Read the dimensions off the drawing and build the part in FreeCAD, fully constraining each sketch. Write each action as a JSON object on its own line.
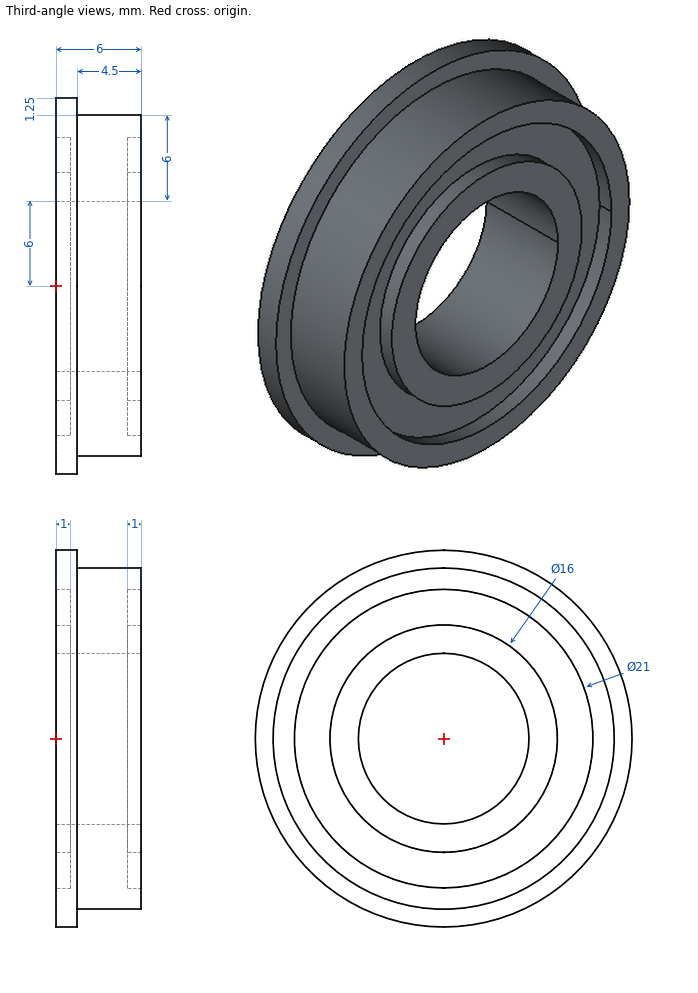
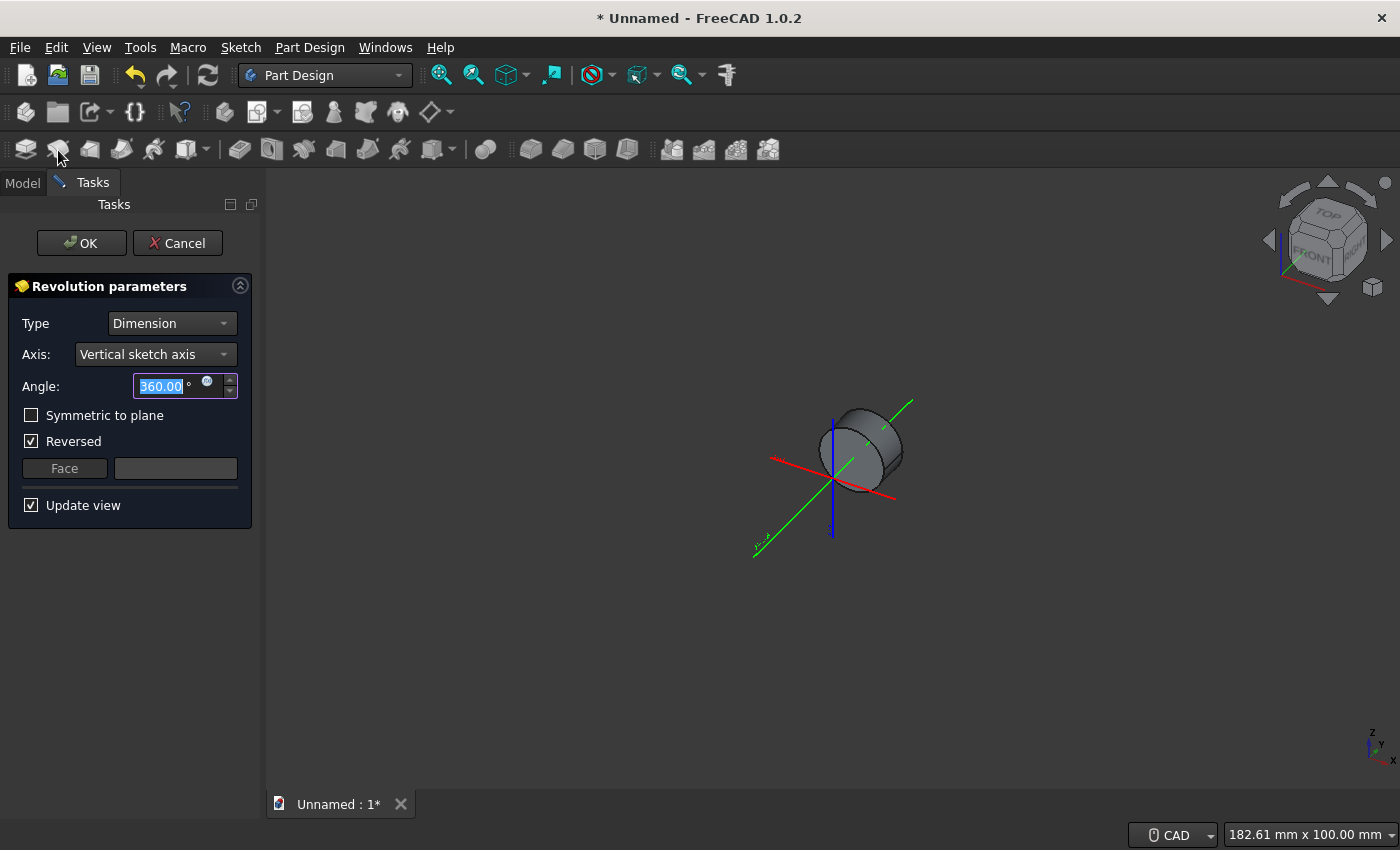
{"action": "left_click", "coordinate": [156, 354]}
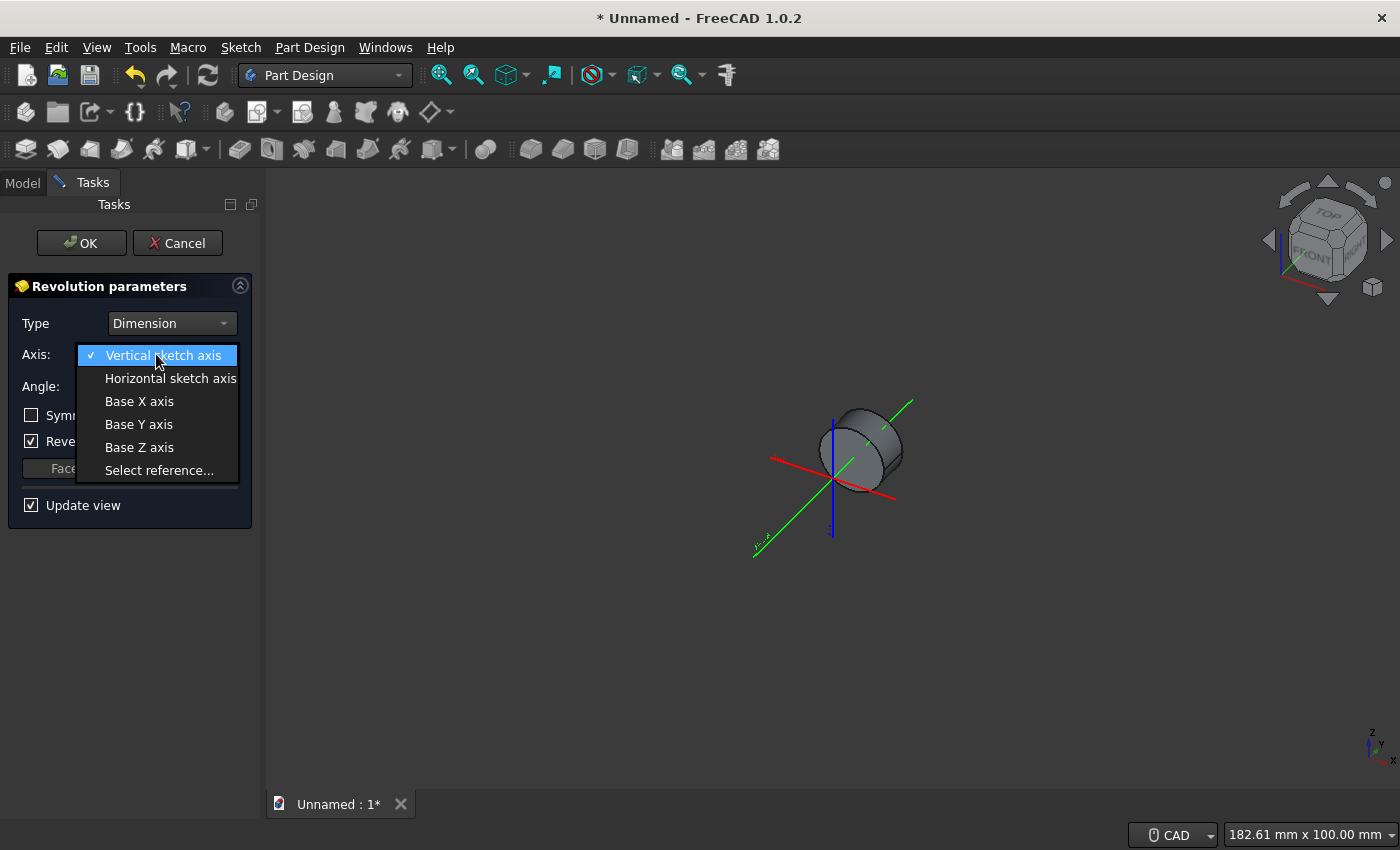
{"action": "left_click", "coordinate": [156, 378]}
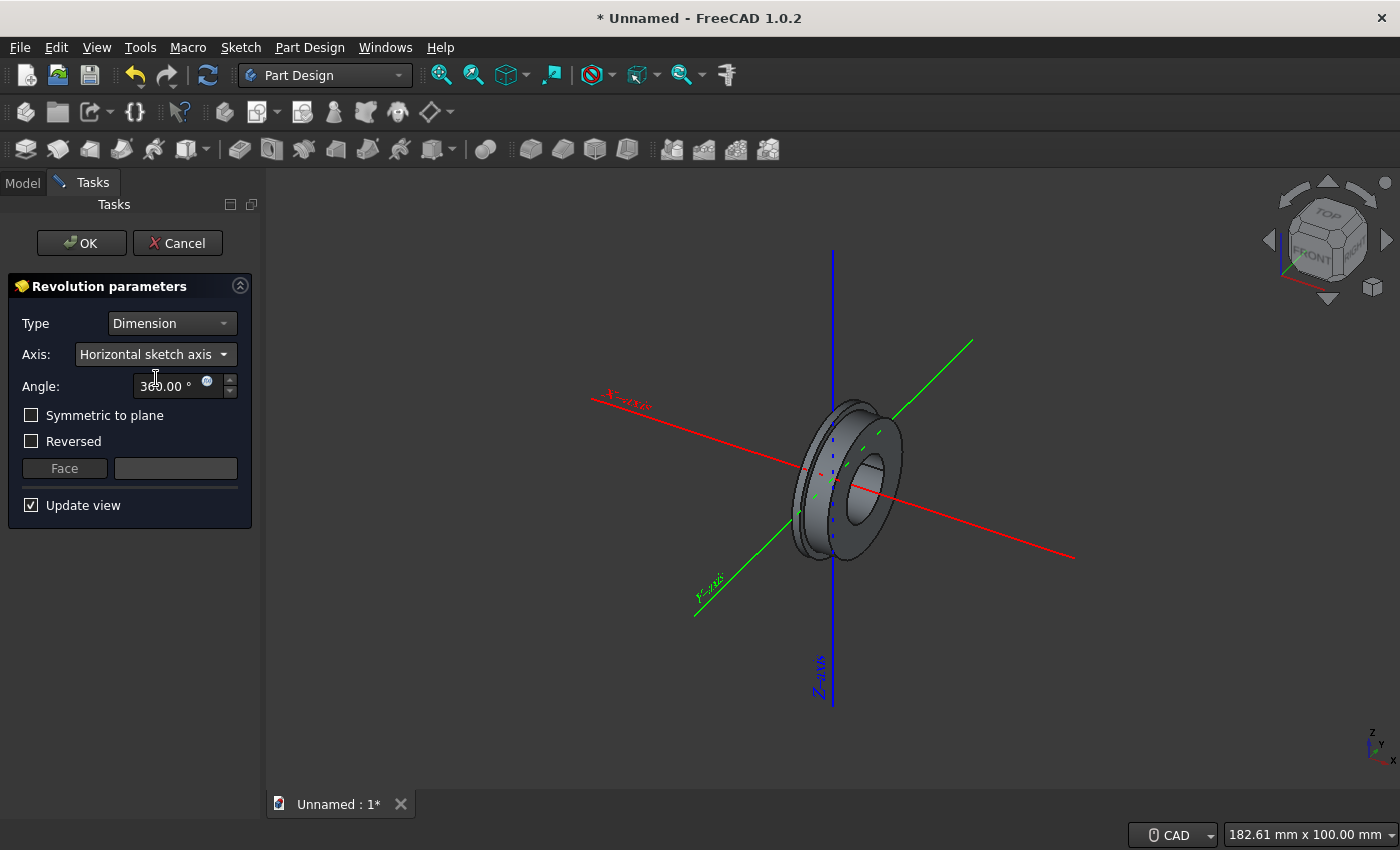
{"action": "left_click", "coordinate": [82, 243]}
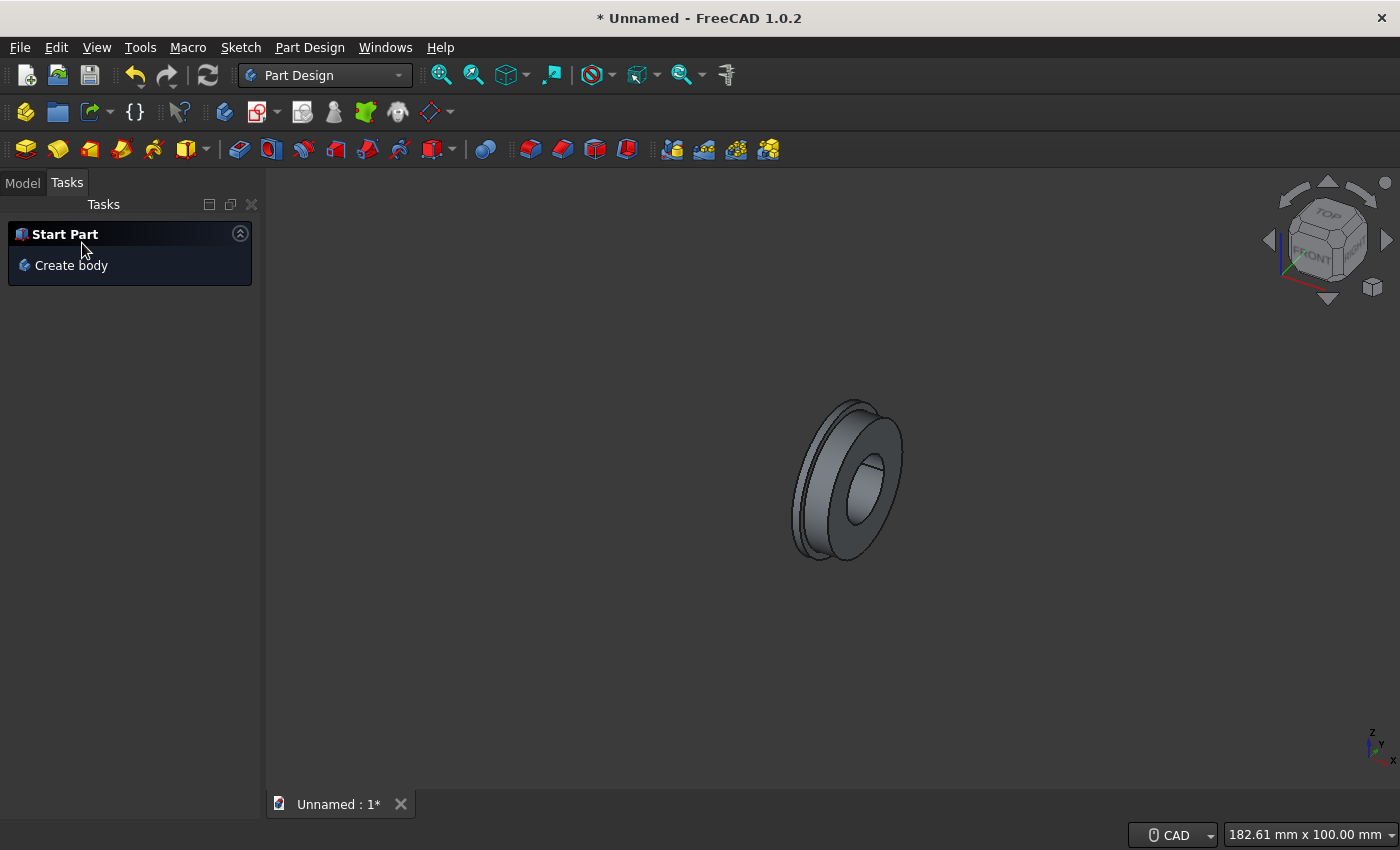
{"action": "left_click", "coordinate": [442, 76]}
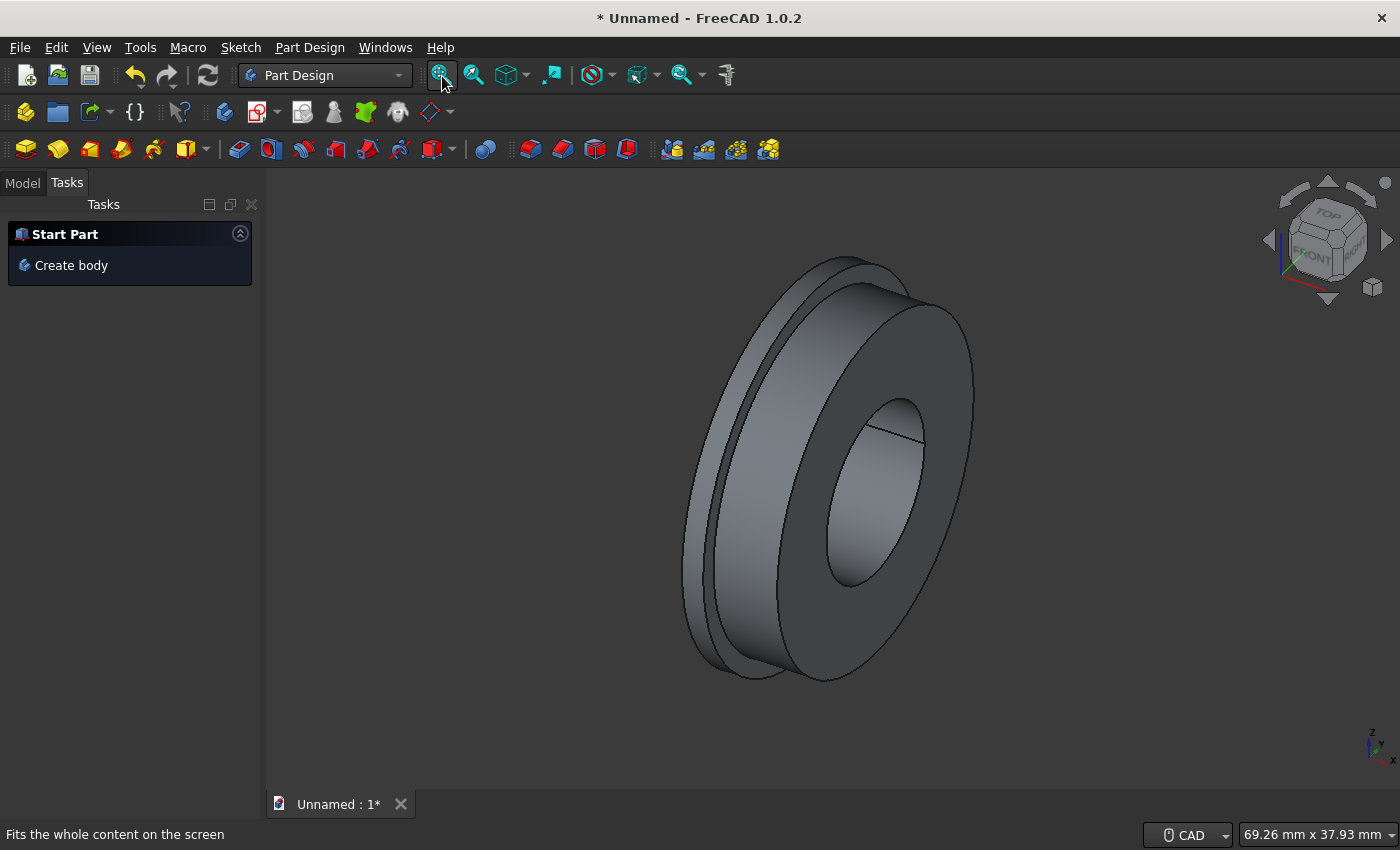
{"action": "left_click", "coordinate": [932, 344]}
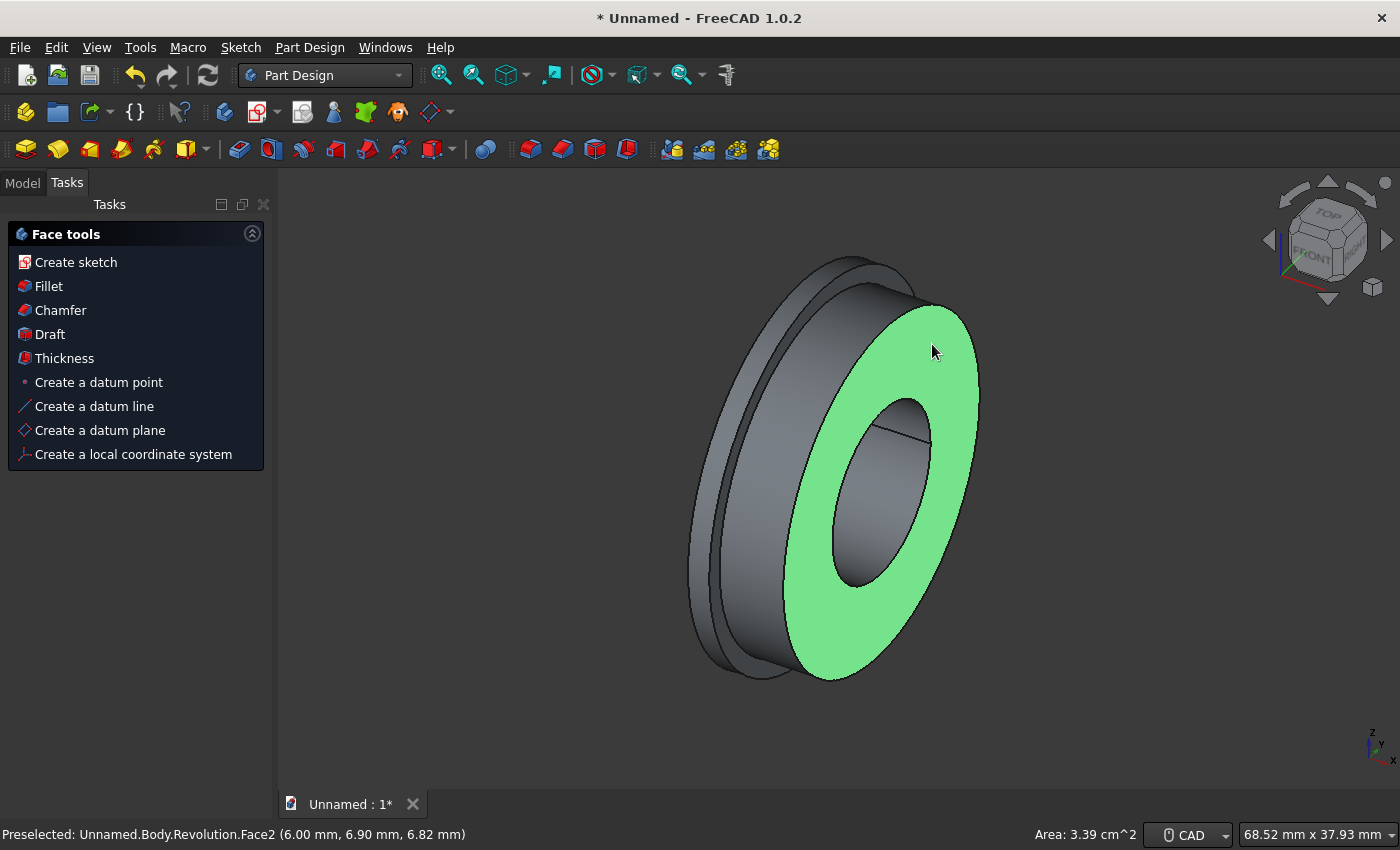
{"action": "left_click", "coordinate": [258, 112]}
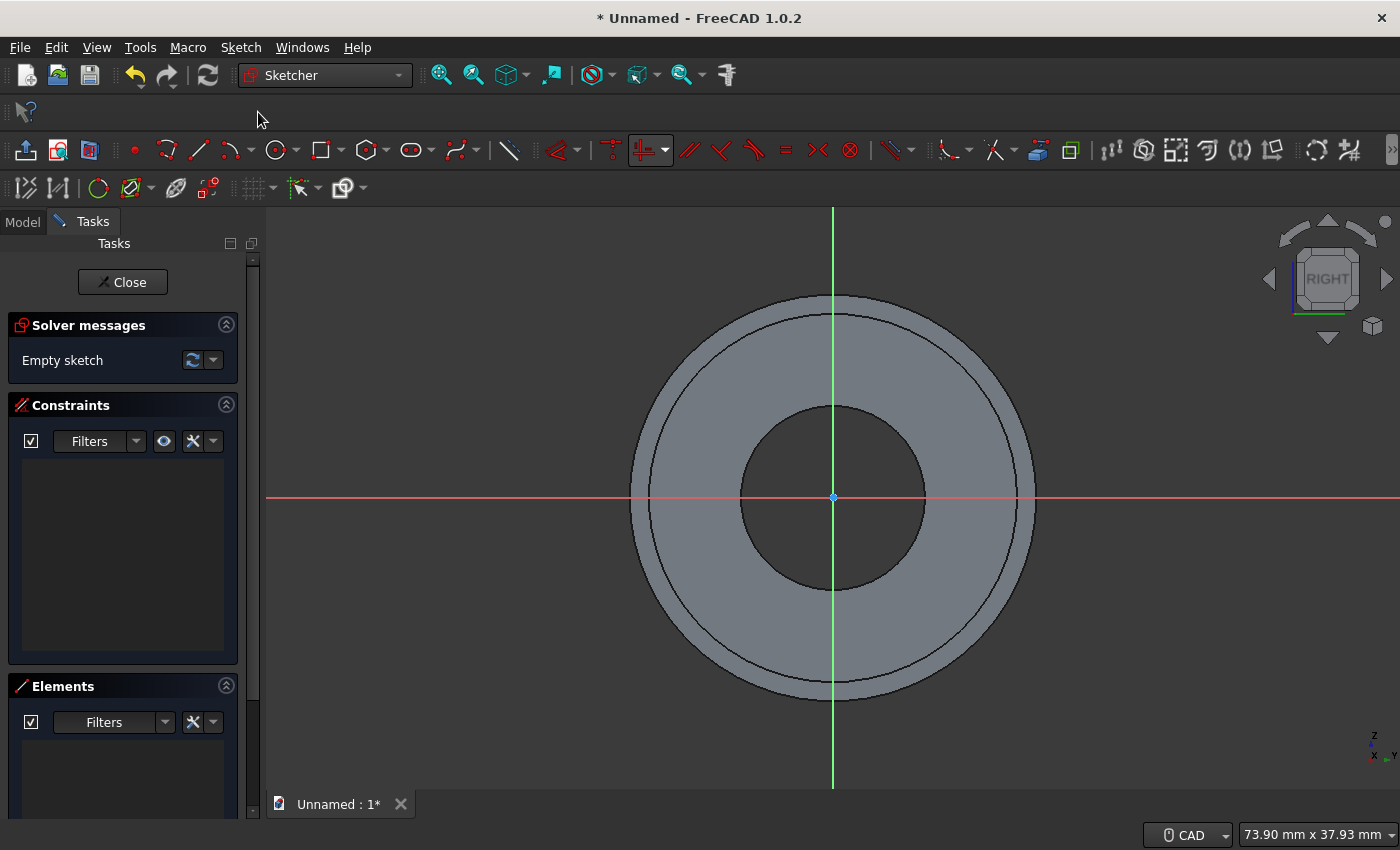
{"action": "key", "text": "g c"}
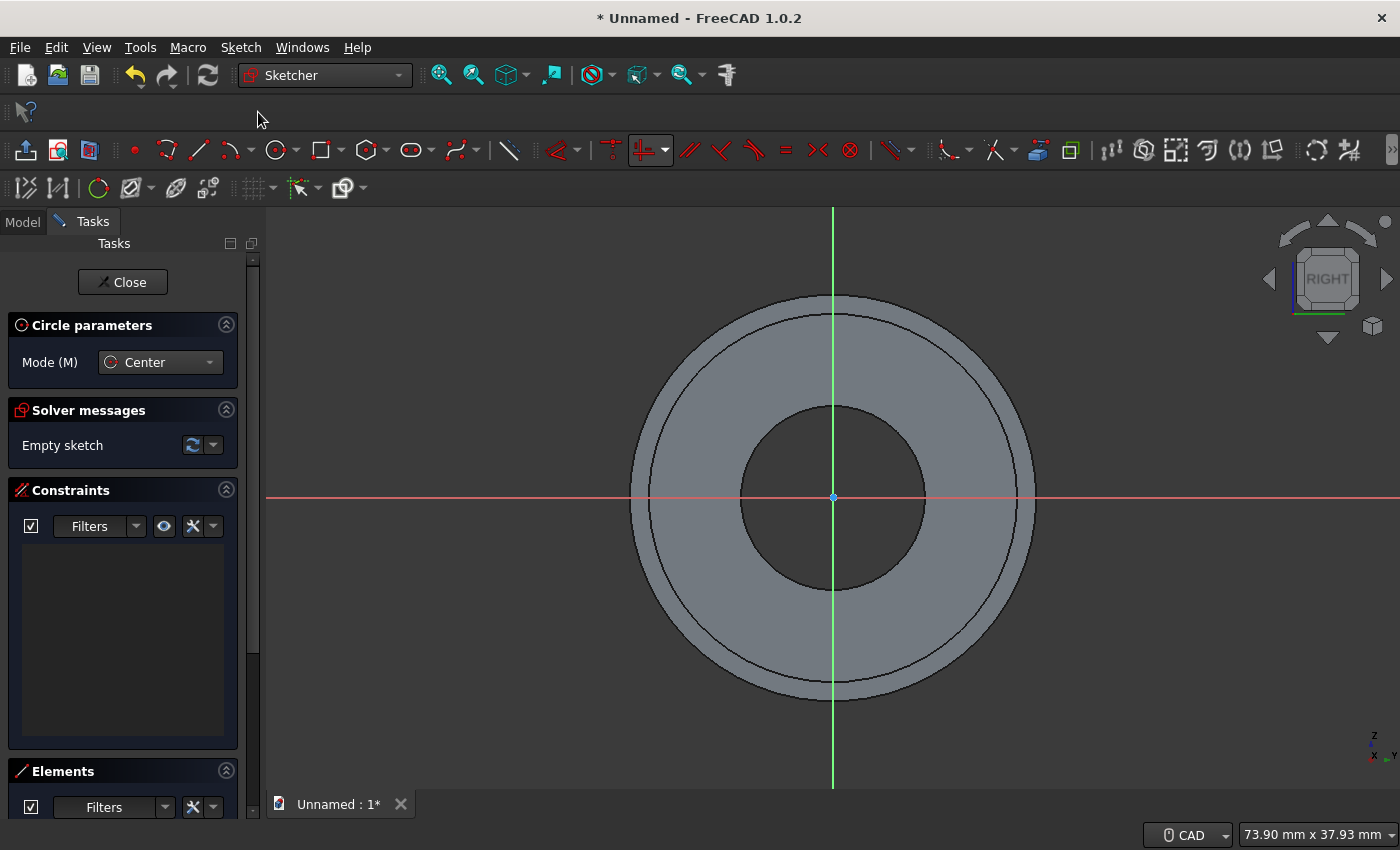
{"action": "left_click", "coordinate": [833, 498]}
{"action": "mouse_move", "coordinate": [947, 384]}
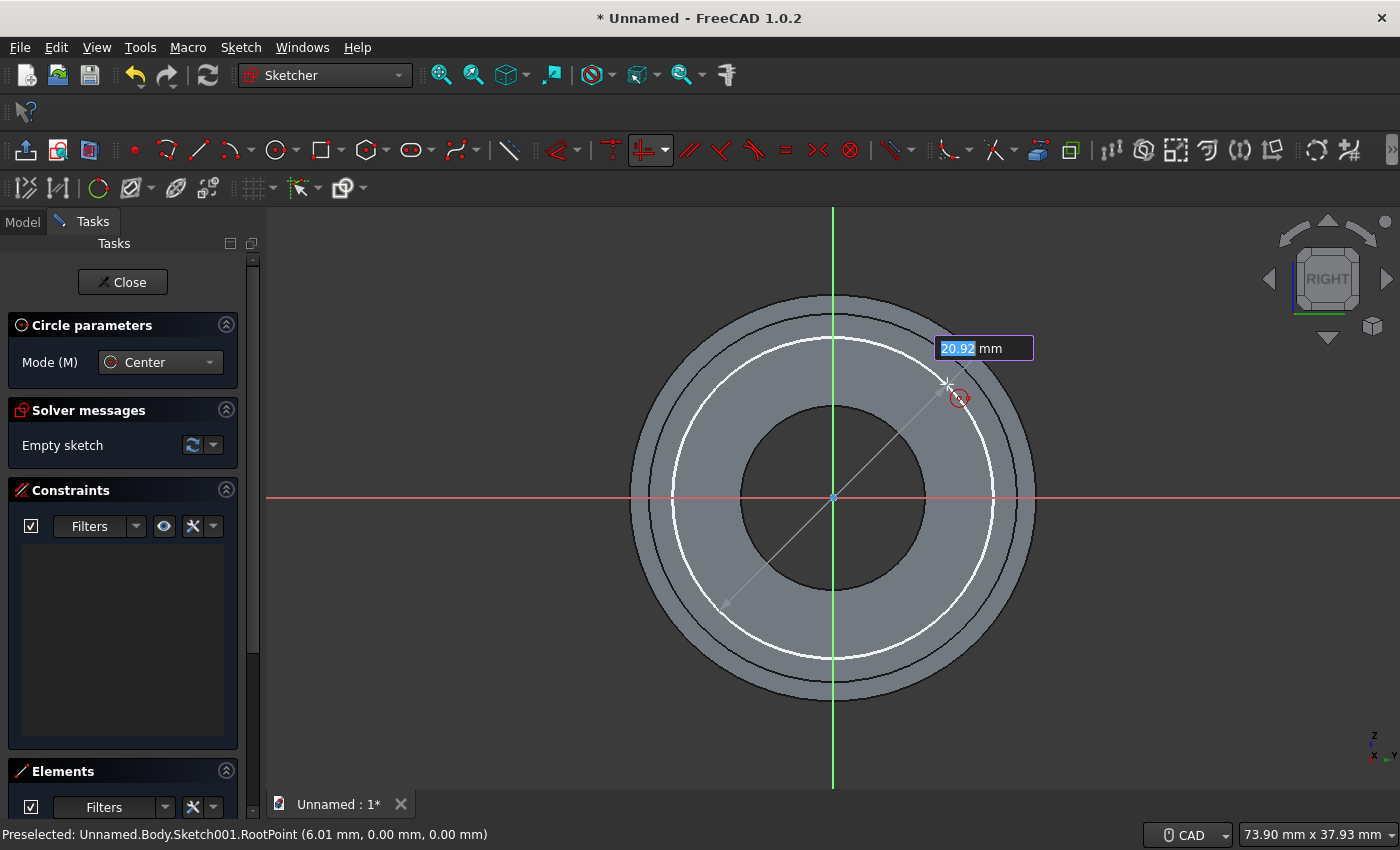
{"action": "type", "text": "21"}
{"action": "key", "text": "Return"}